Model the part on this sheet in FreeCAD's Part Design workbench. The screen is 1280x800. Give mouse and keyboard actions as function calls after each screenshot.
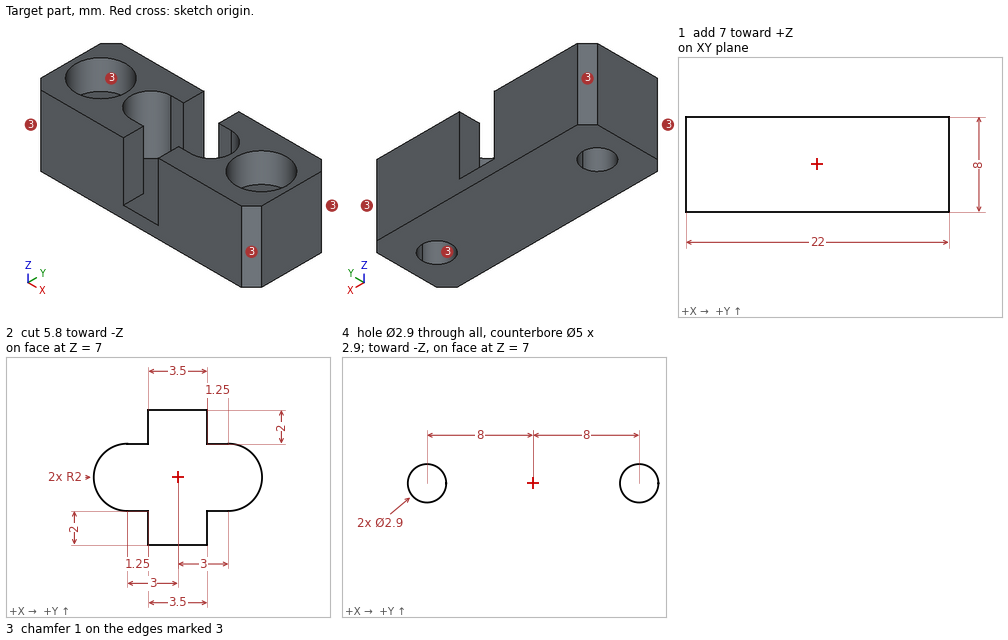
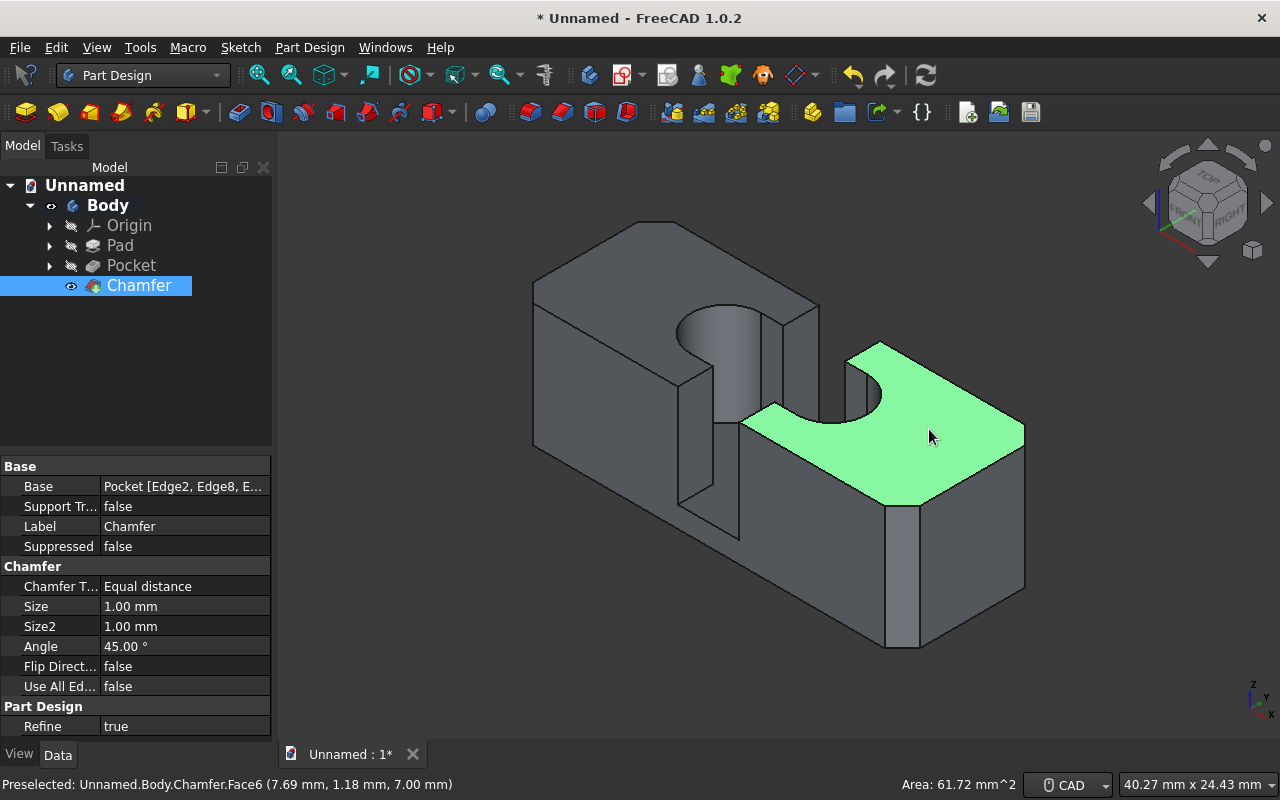
click(622, 76)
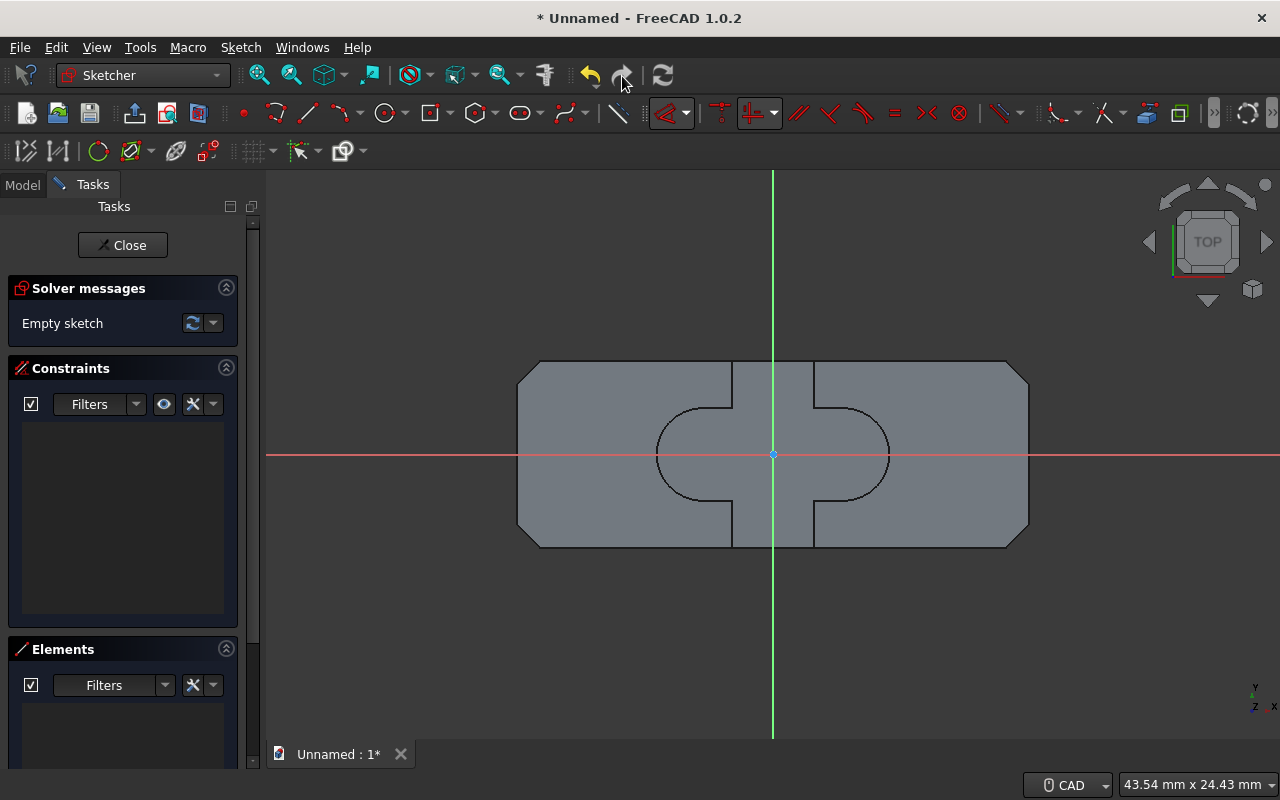
click(386, 114)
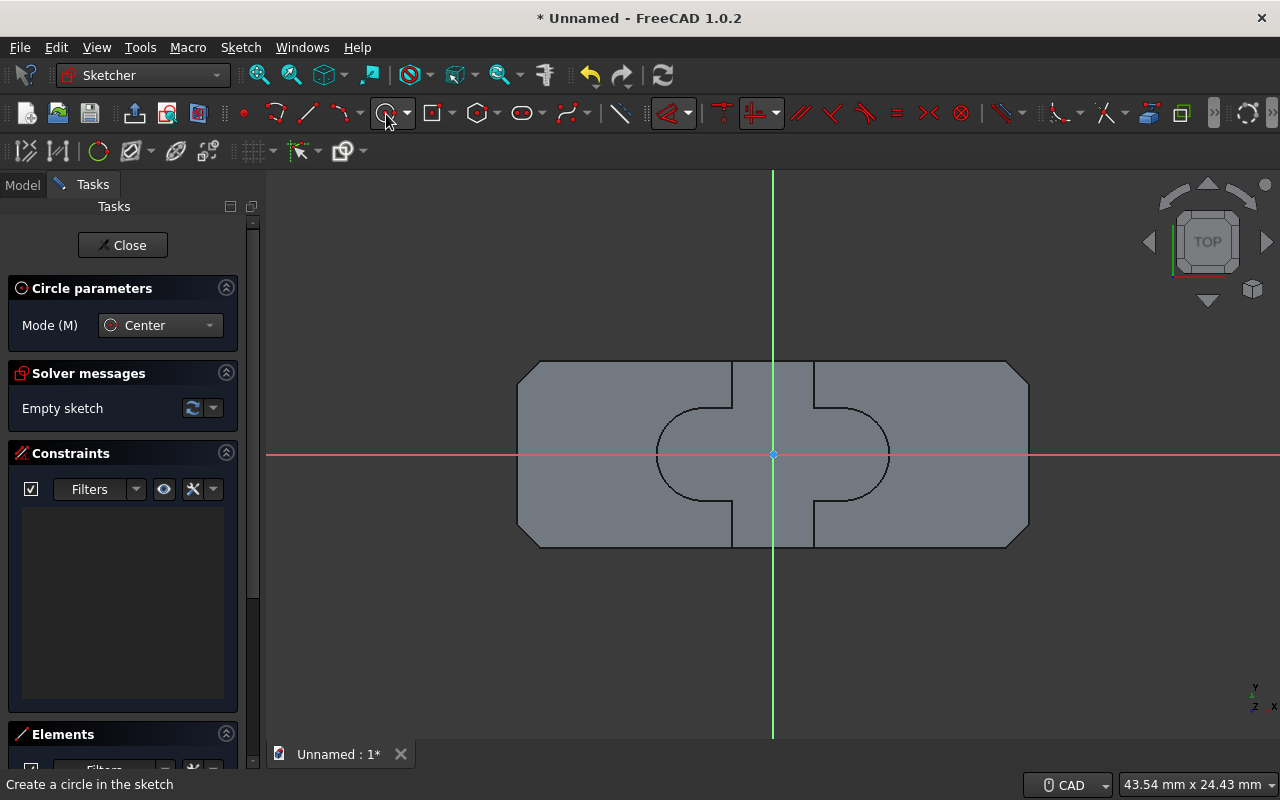
click(587, 455)
click(611, 431)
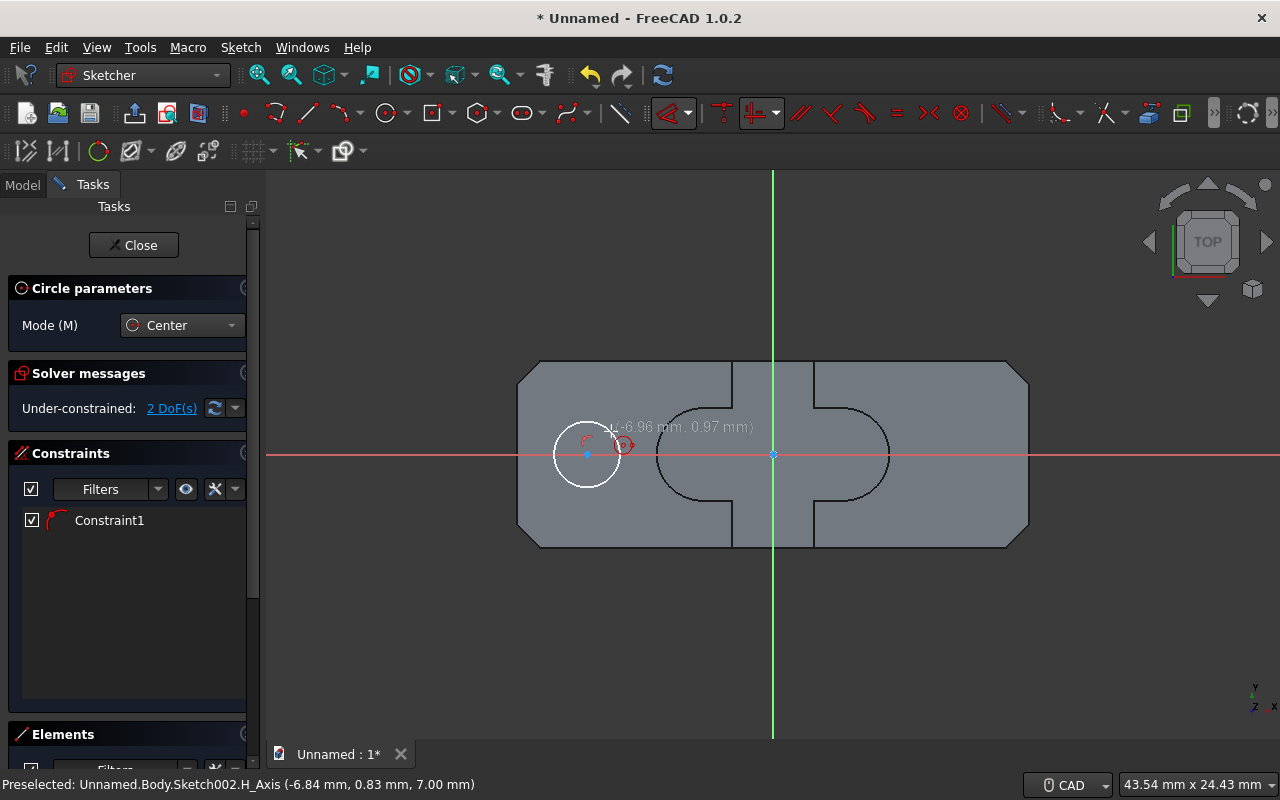
click(959, 455)
click(983, 431)
key(Escape)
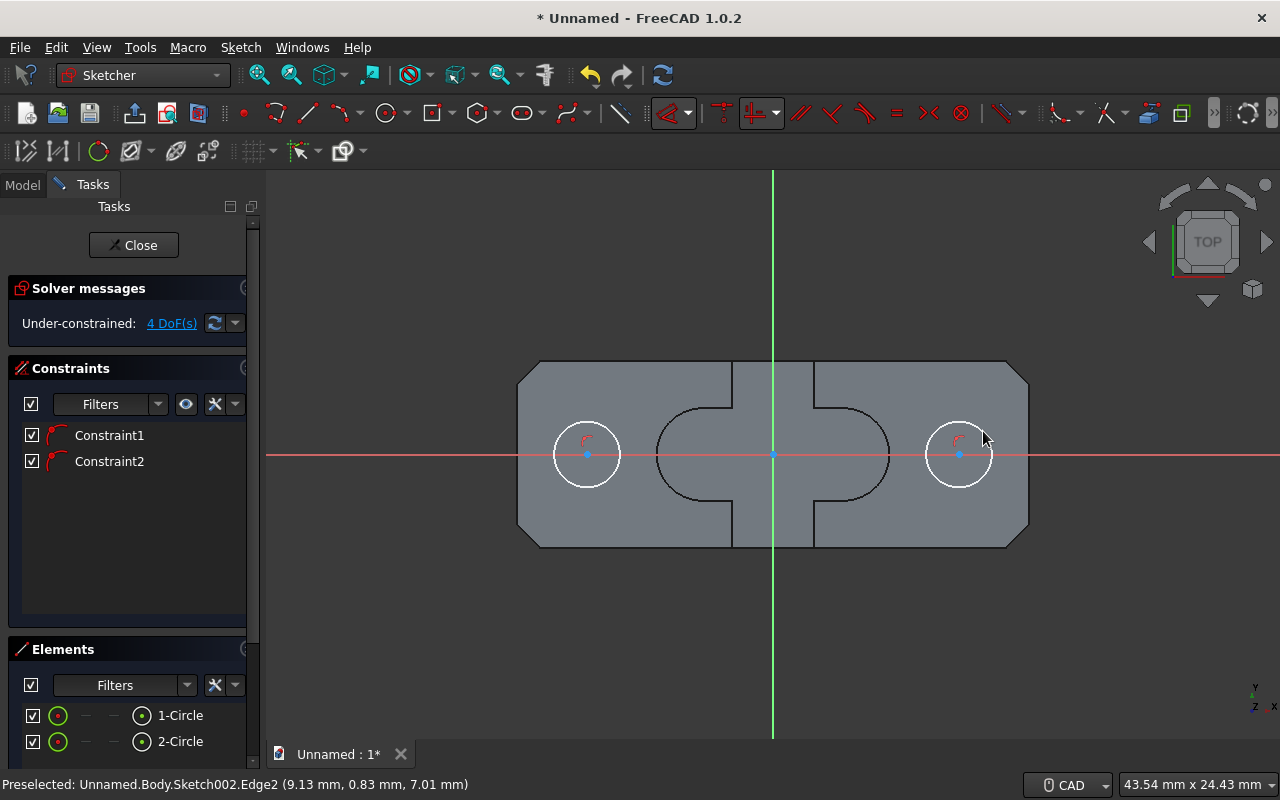
click(610, 431)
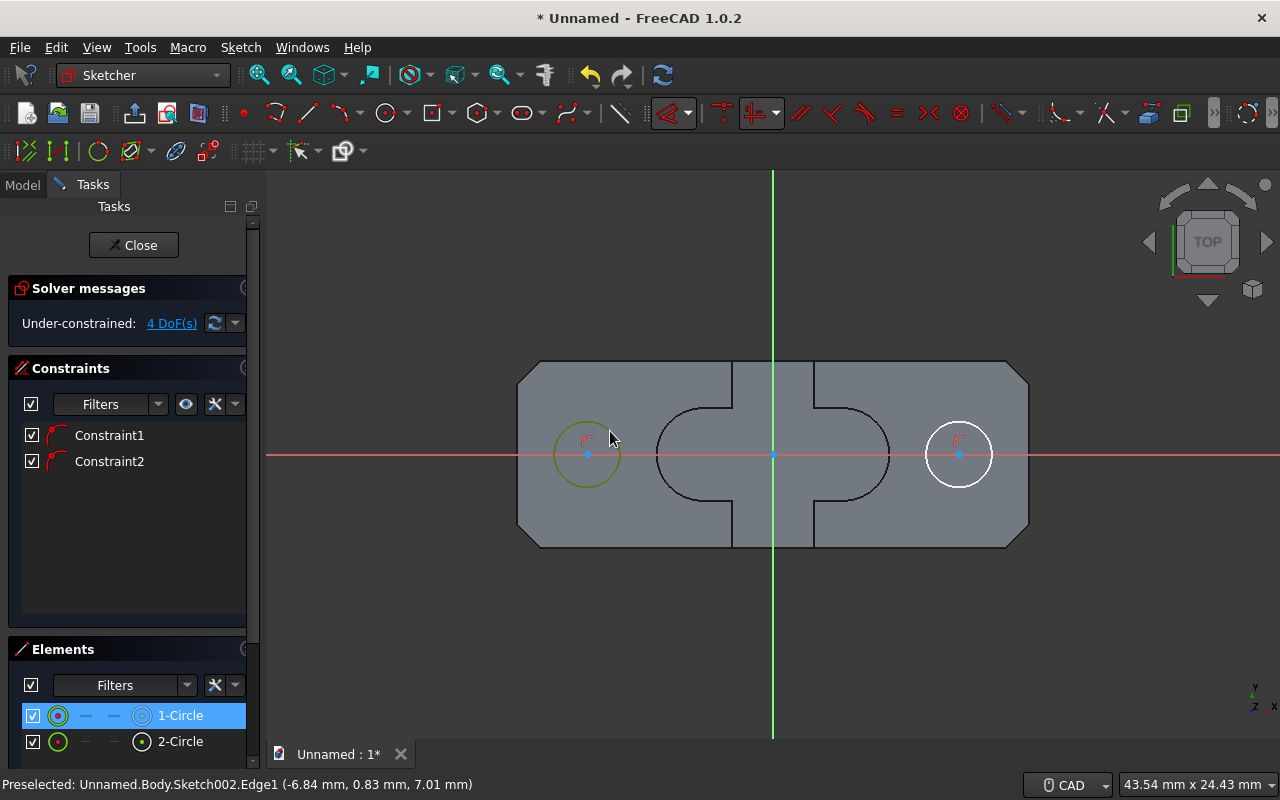
click(982, 431)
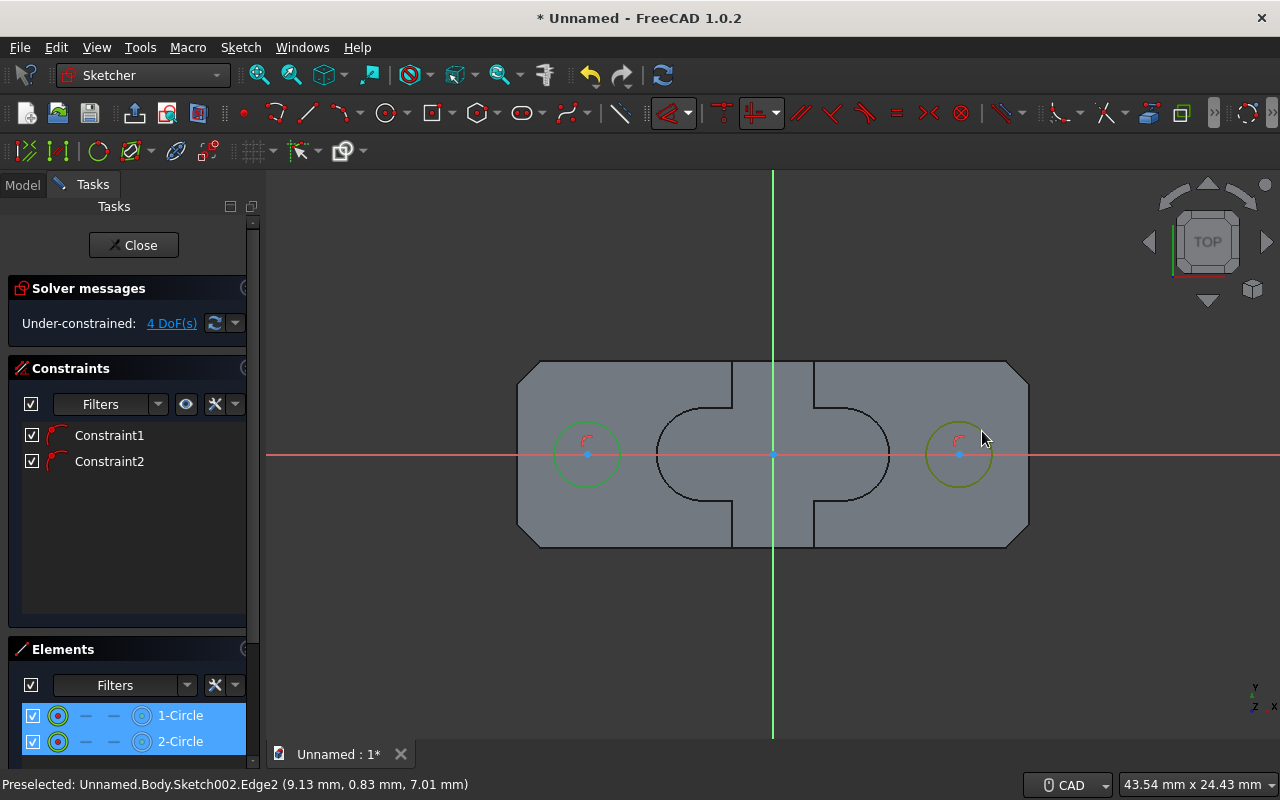
click(898, 114)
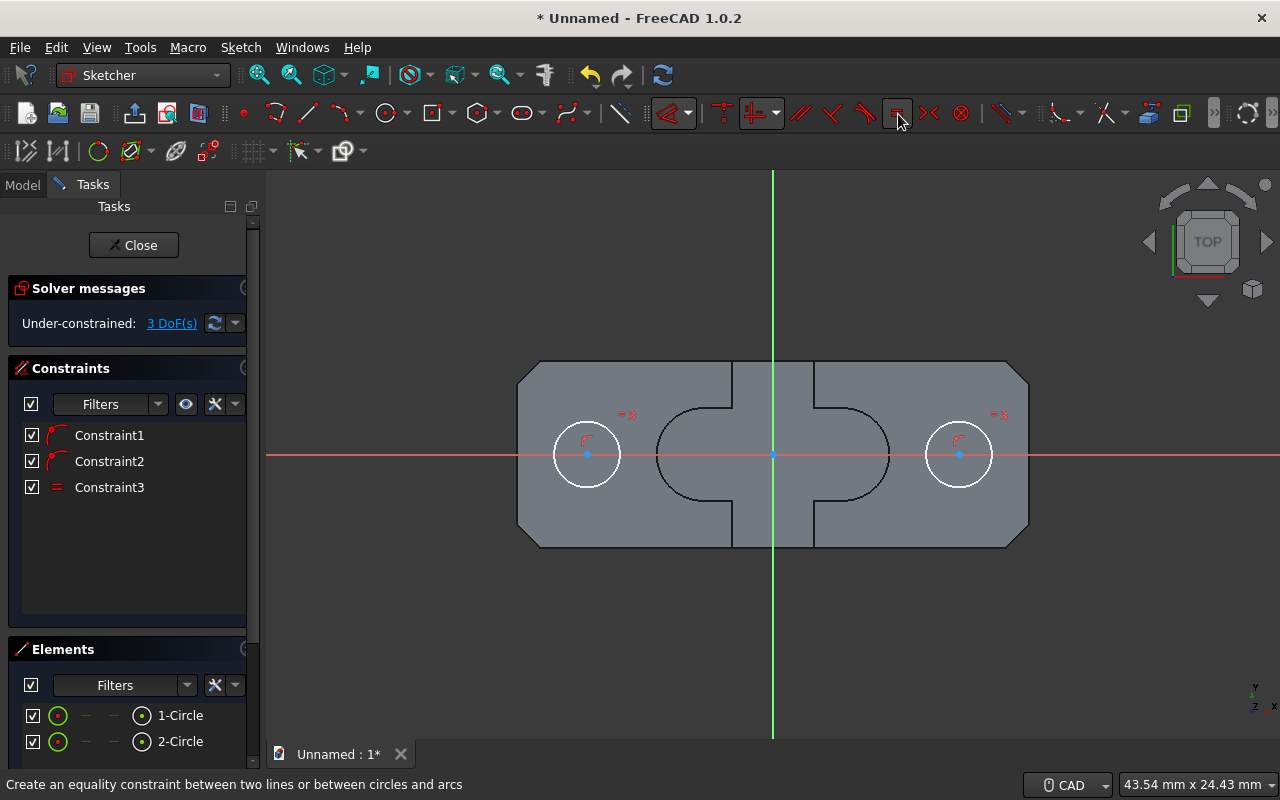
click(610, 431)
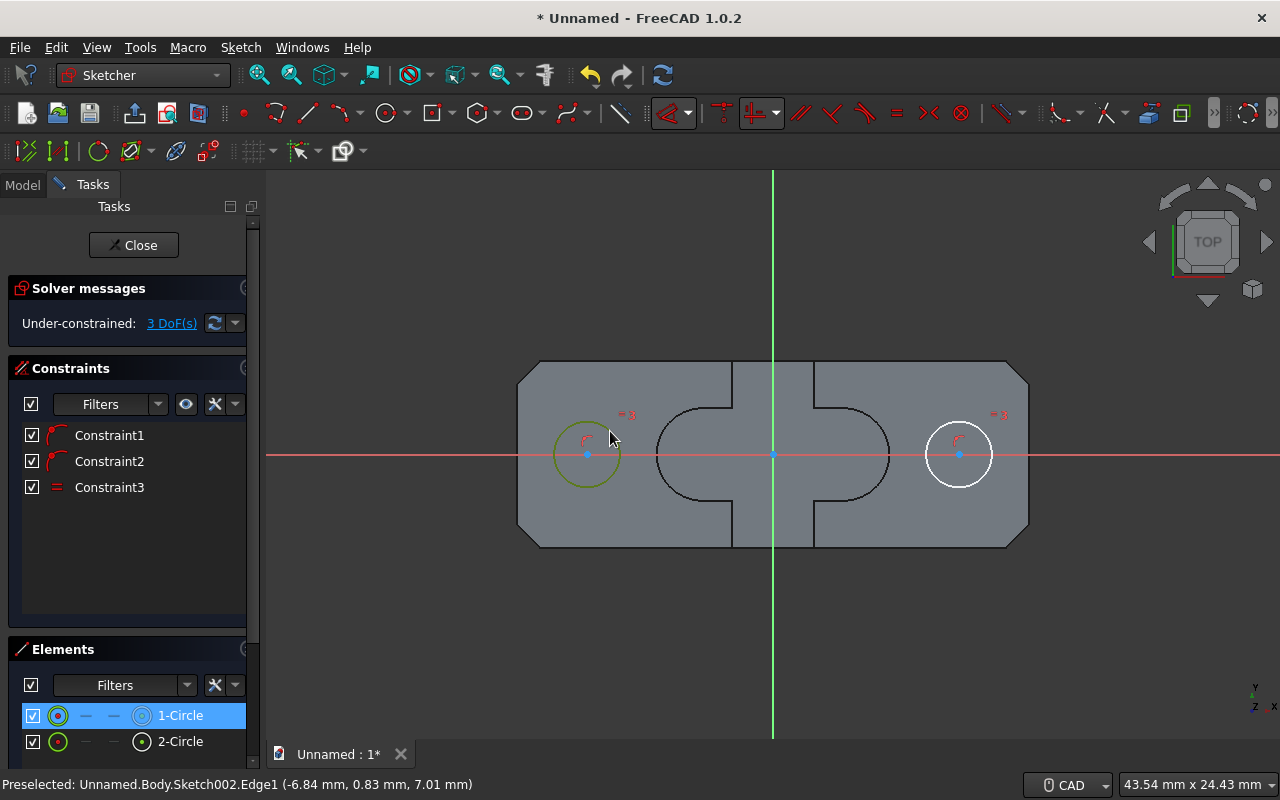
click(690, 114)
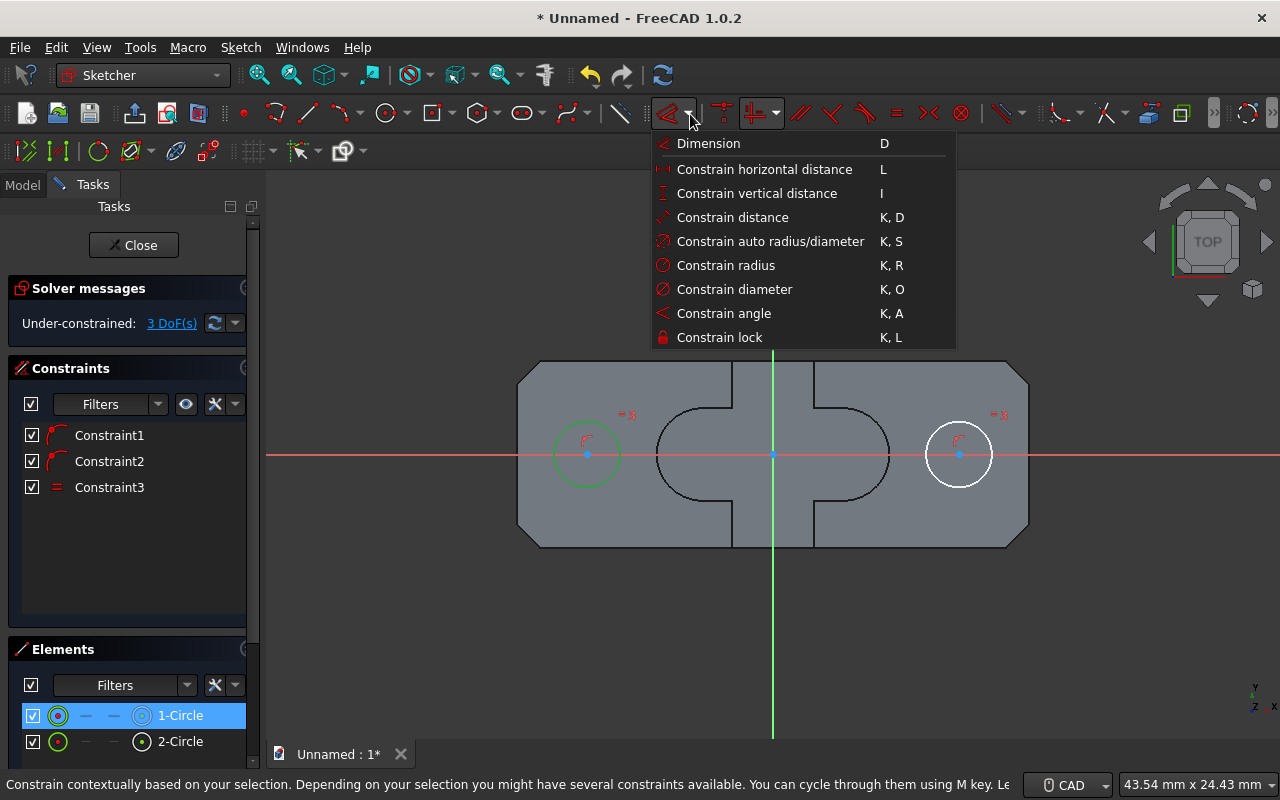
click(804, 289)